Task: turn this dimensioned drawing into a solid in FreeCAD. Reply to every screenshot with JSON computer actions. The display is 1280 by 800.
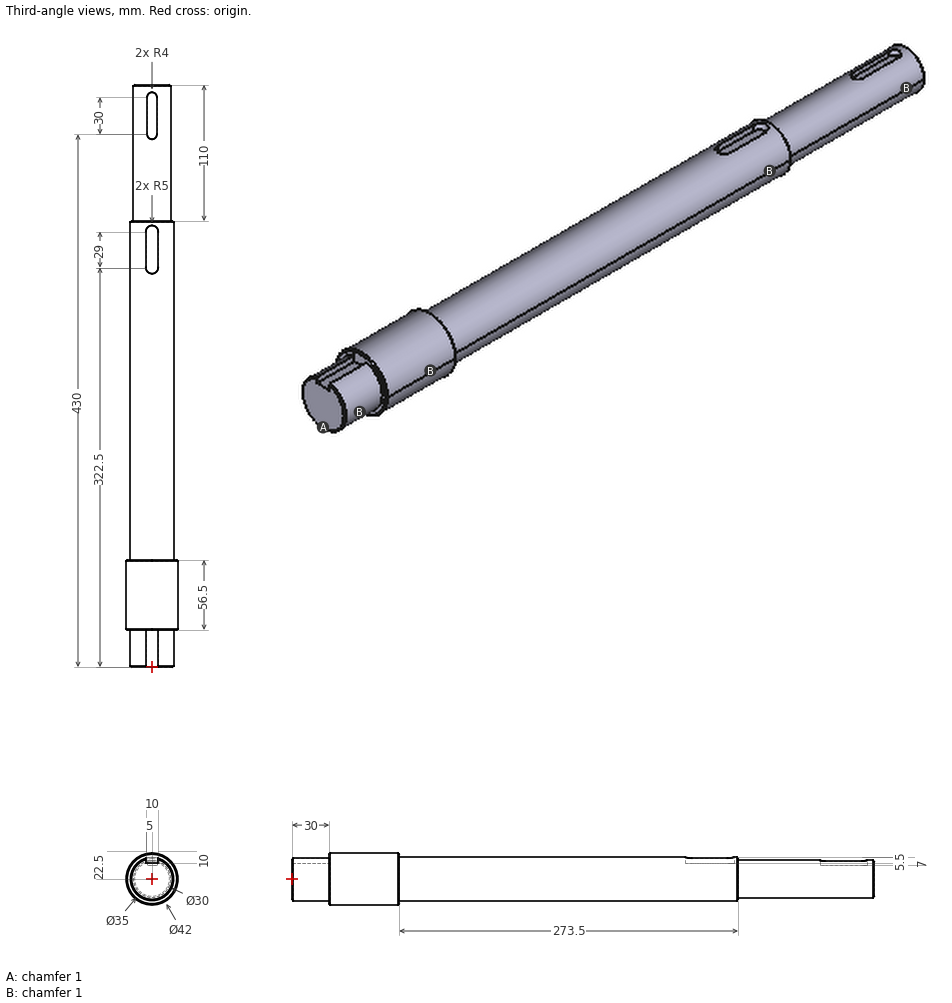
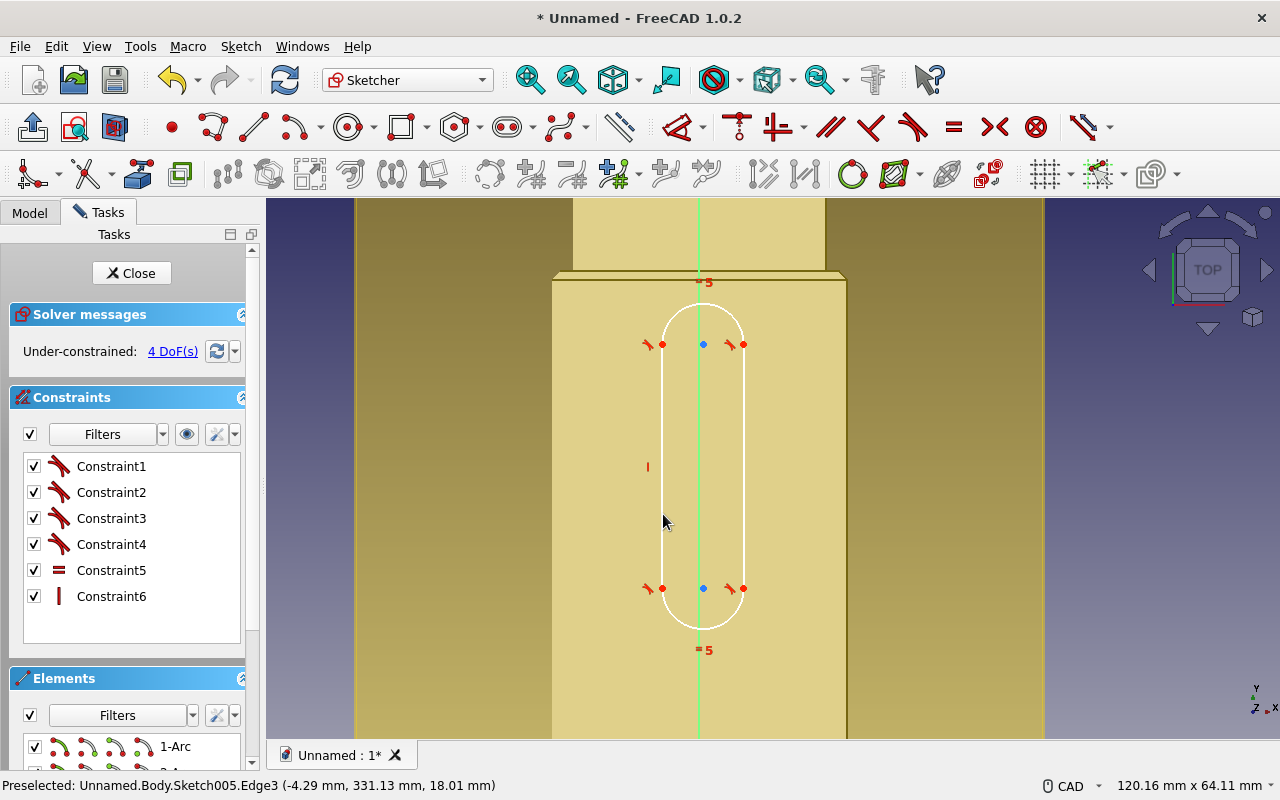
{"action": "left_click", "coordinate": [703, 588]}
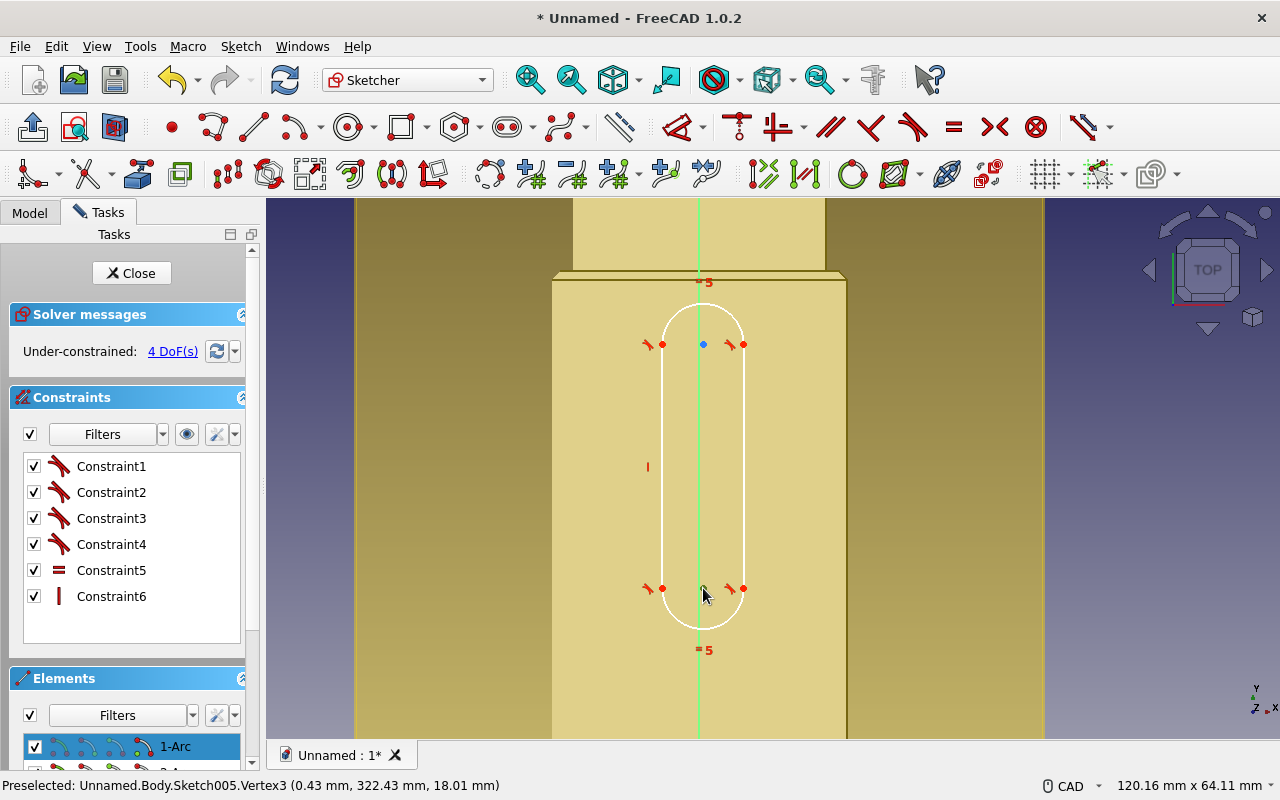
{"action": "left_click", "coordinate": [699, 676]}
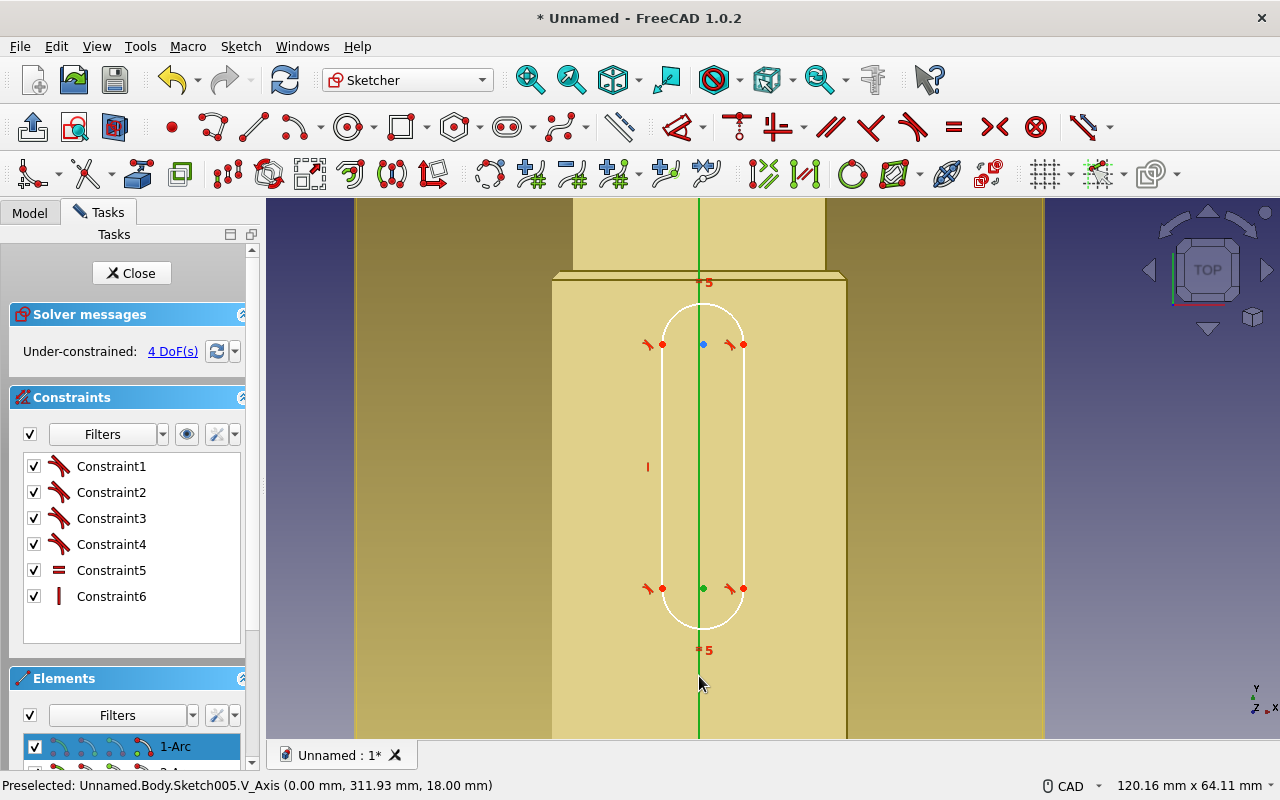
{"action": "left_click", "coordinate": [737, 128]}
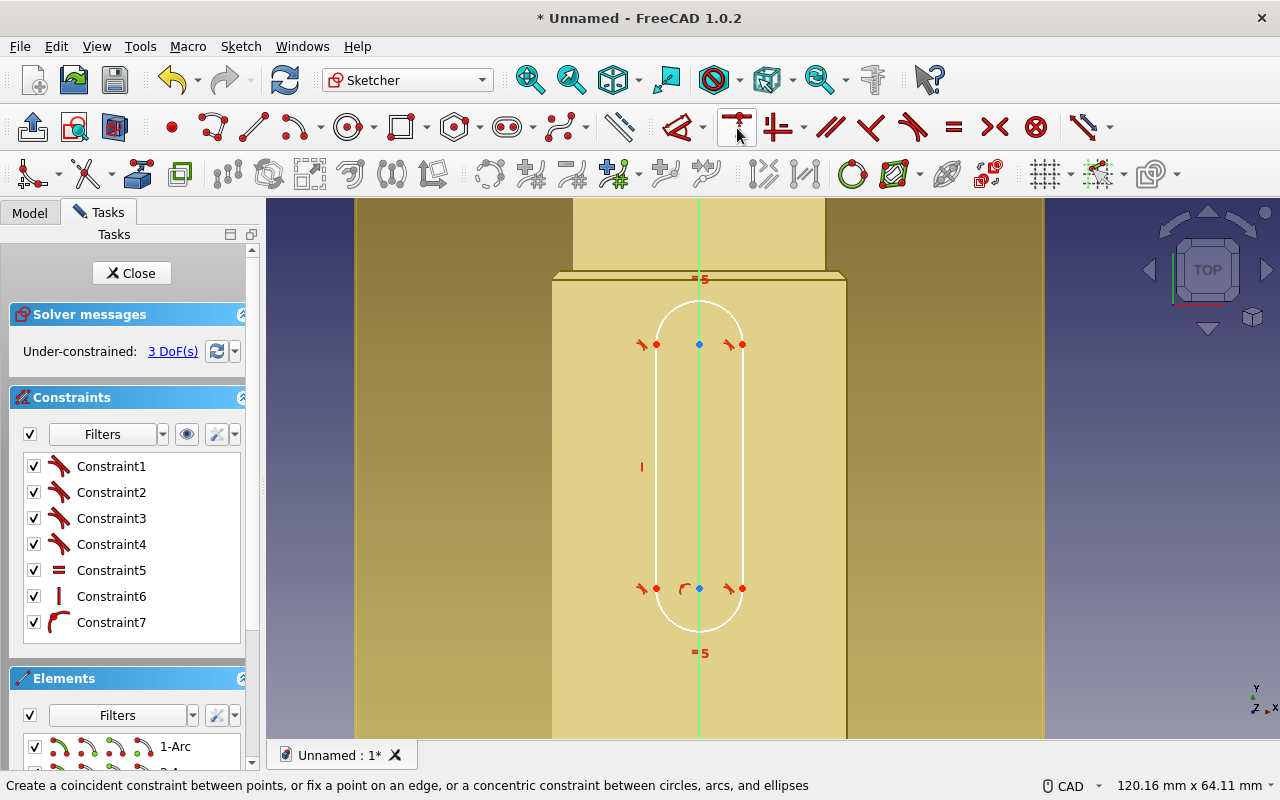
{"action": "left_click", "coordinate": [676, 128]}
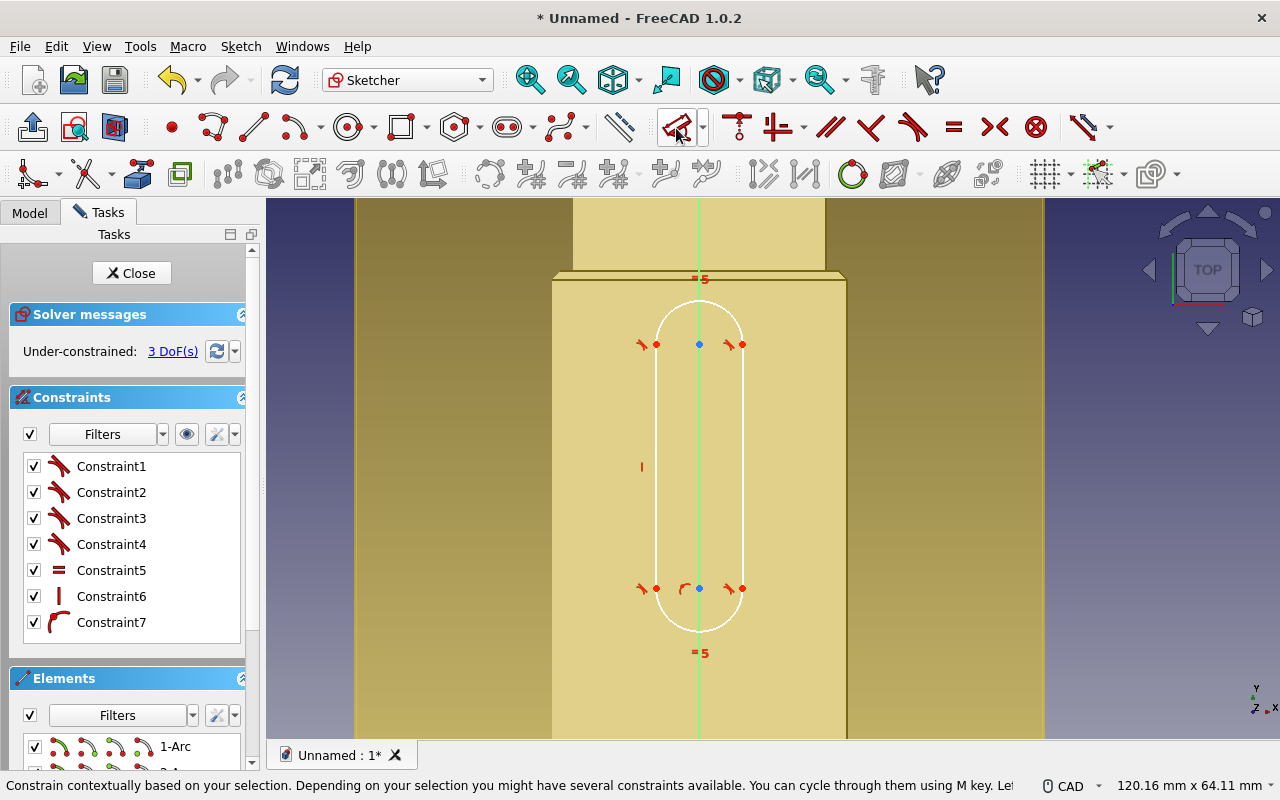
{"action": "left_click", "coordinate": [674, 623]}
{"action": "left_click", "coordinate": [655, 649]}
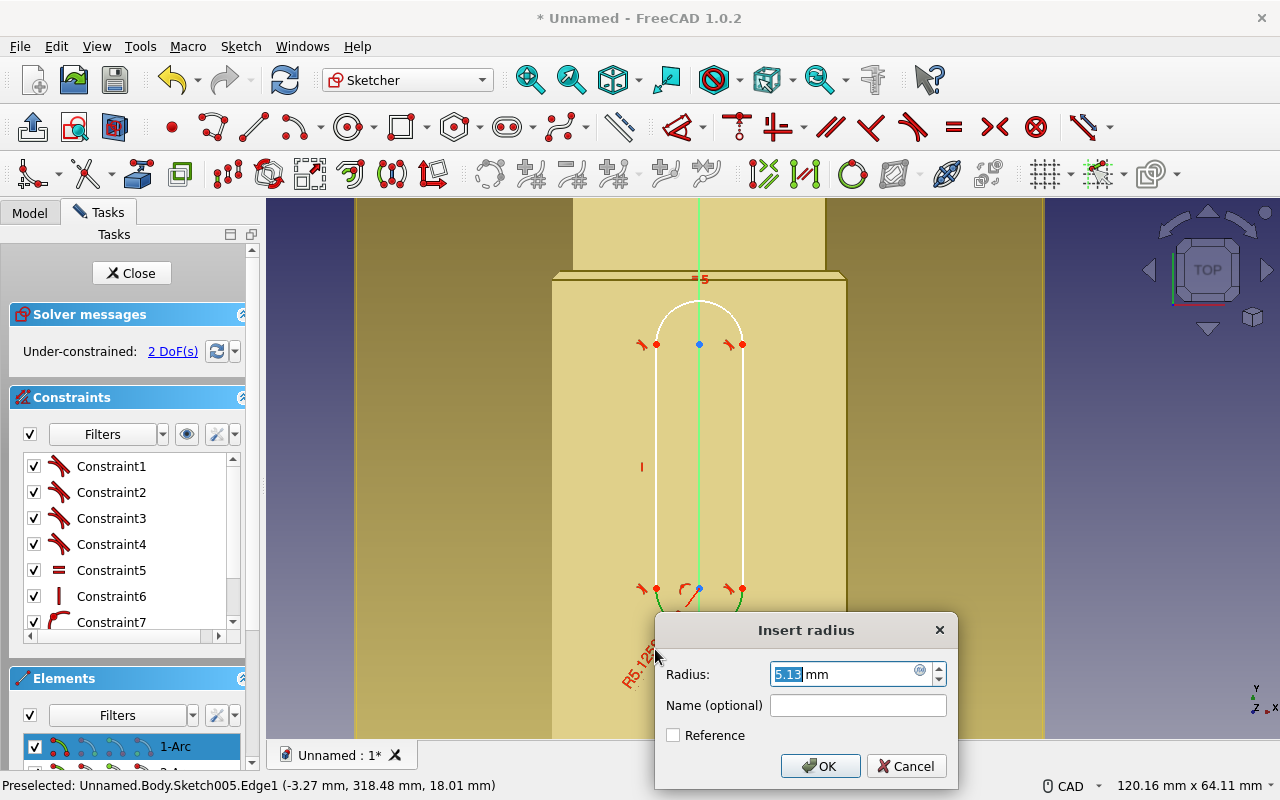
{"action": "type", "text": "5"}
{"action": "key", "text": "Return"}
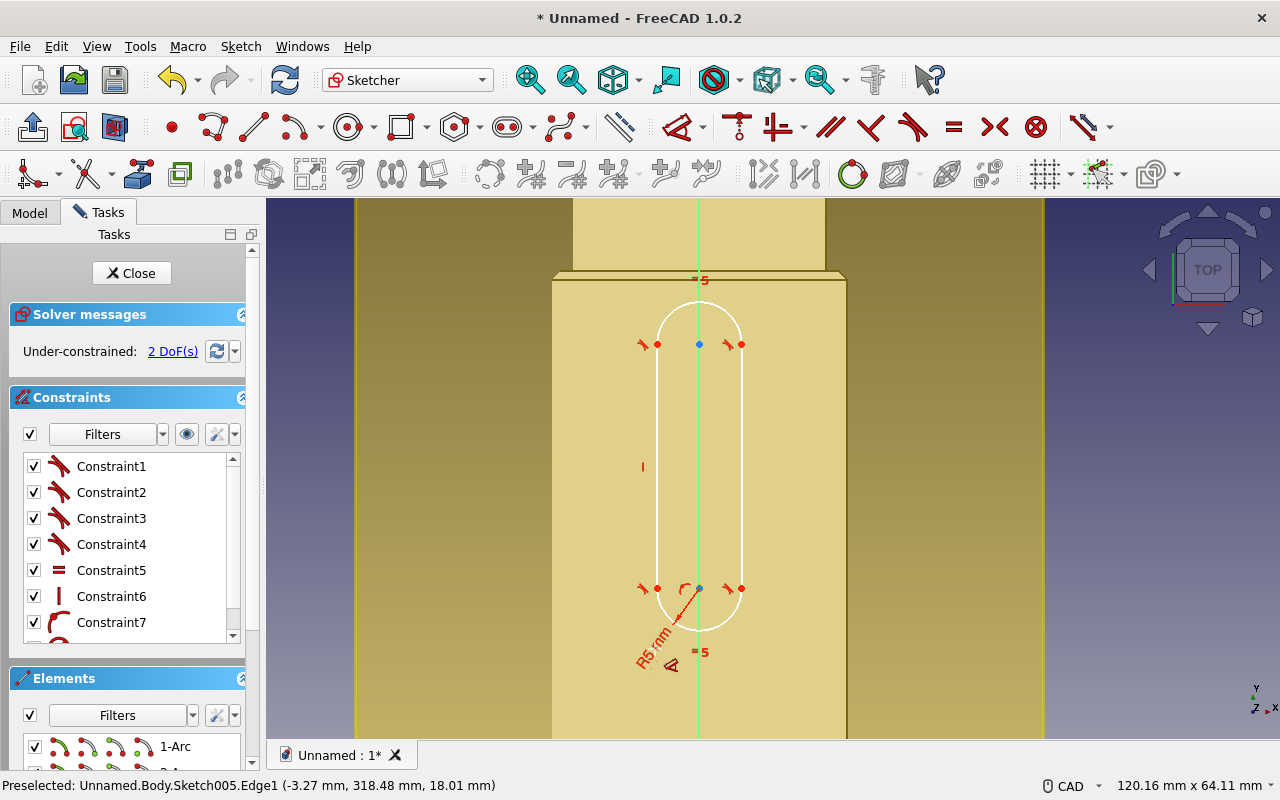
{"action": "left_click", "coordinate": [657, 515]}
{"action": "left_click", "coordinate": [623, 466]}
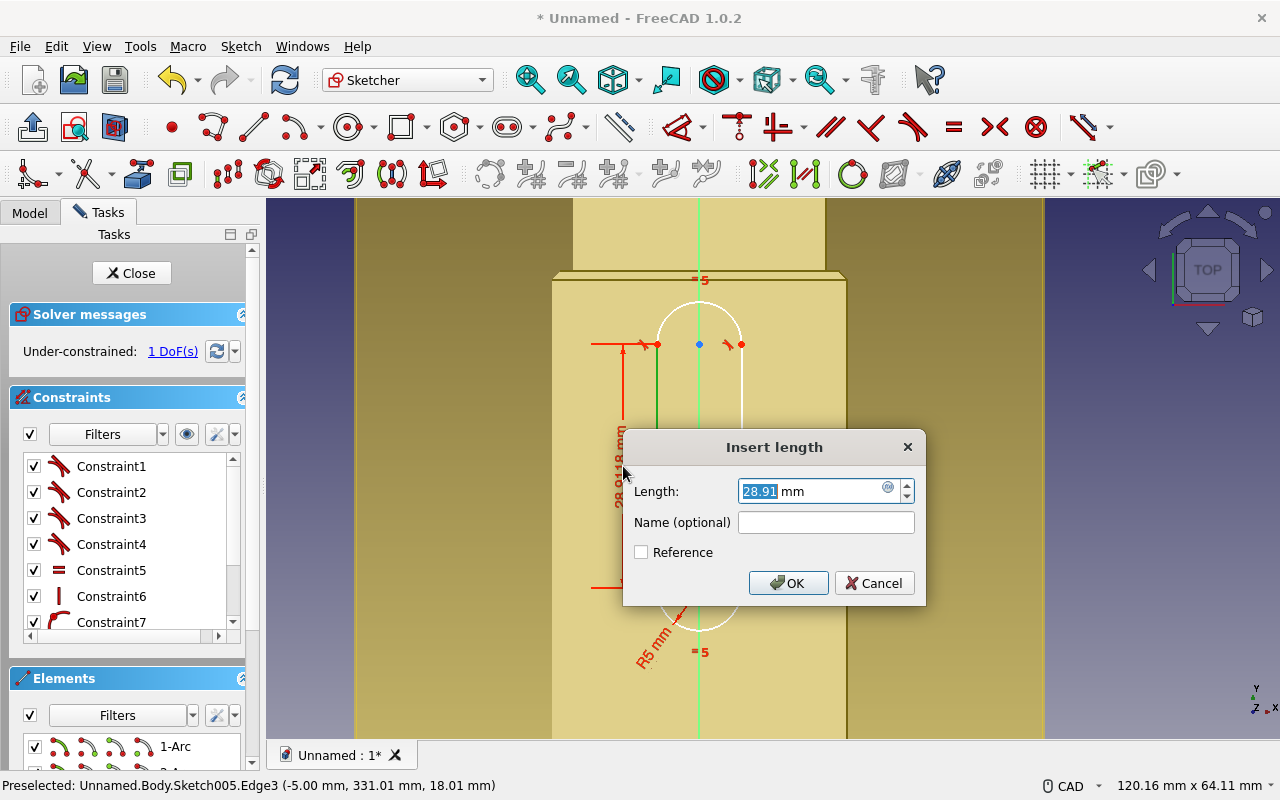
{"action": "type", "text": "29"}
{"action": "key", "text": "Return"}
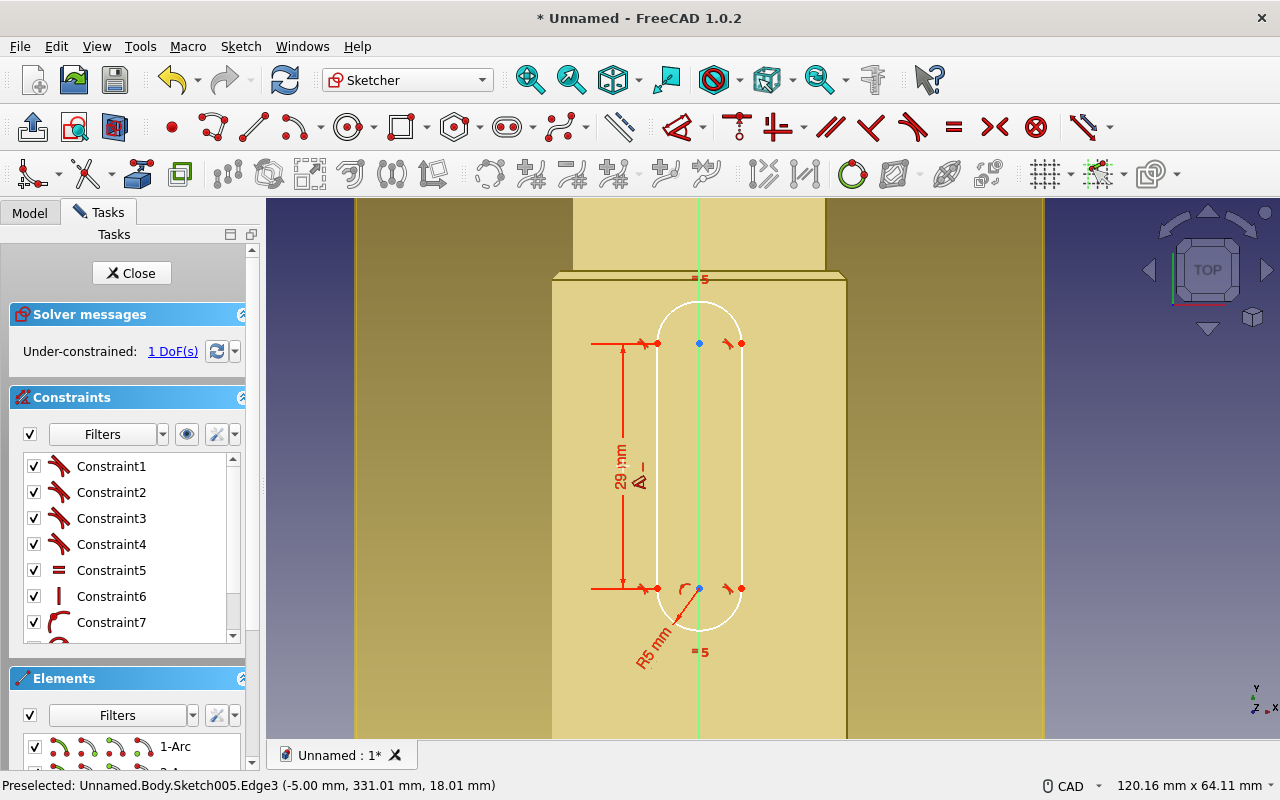
{"action": "left_click", "coordinate": [657, 589]}
{"action": "left_click", "coordinate": [623, 622]}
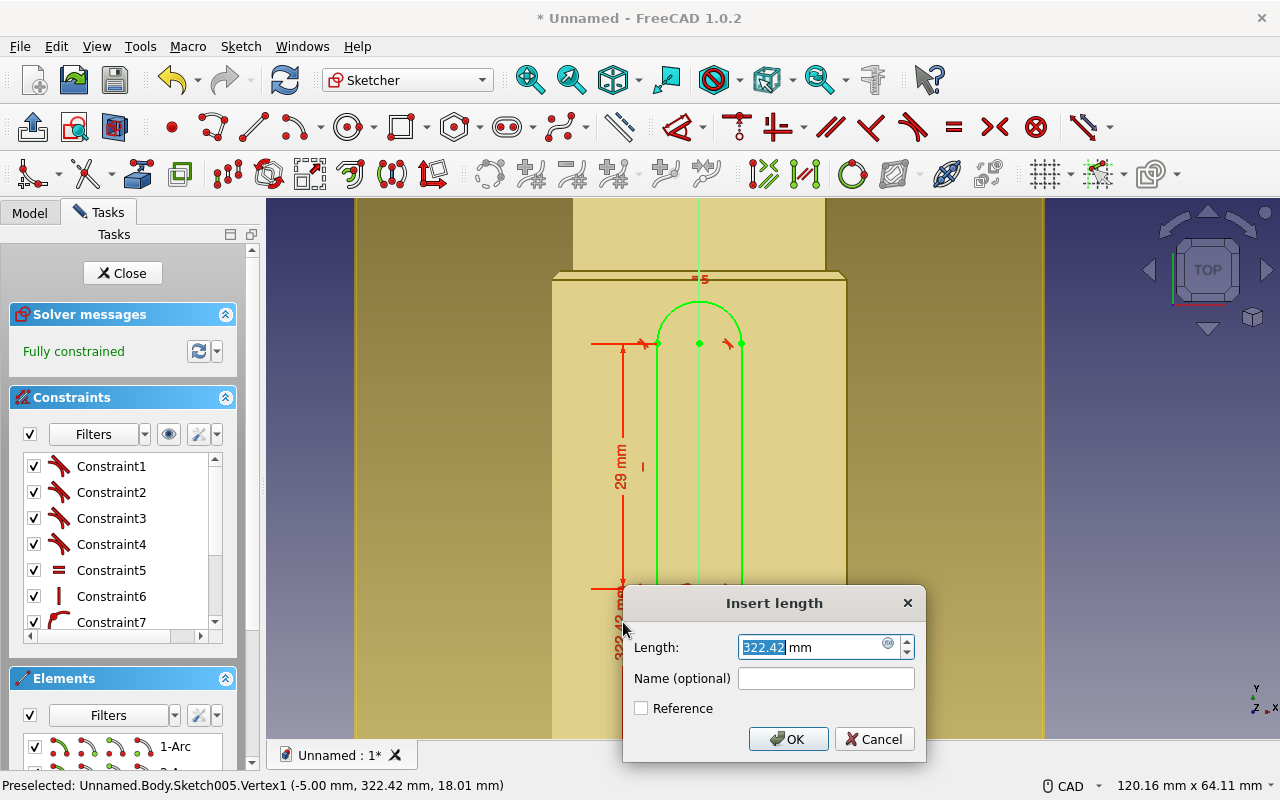
{"action": "type", "text": "322.5"}
{"action": "key", "text": "Return"}
{"action": "key", "text": "Escape"}